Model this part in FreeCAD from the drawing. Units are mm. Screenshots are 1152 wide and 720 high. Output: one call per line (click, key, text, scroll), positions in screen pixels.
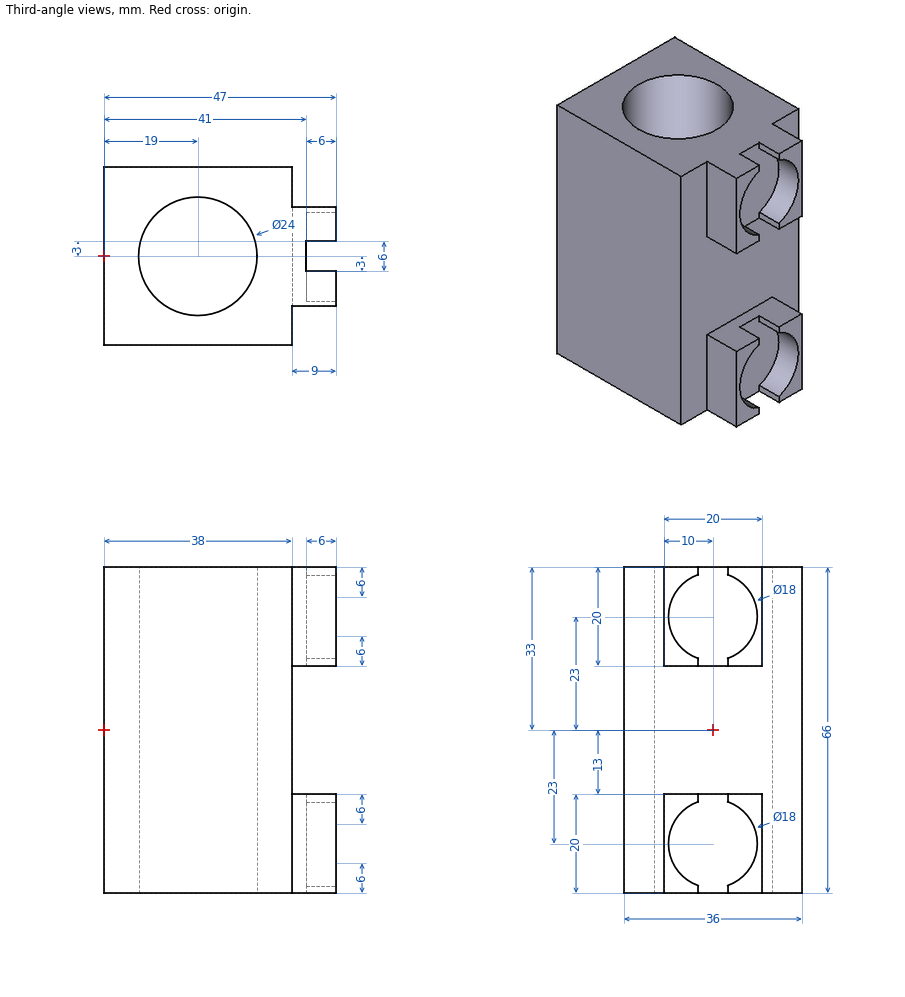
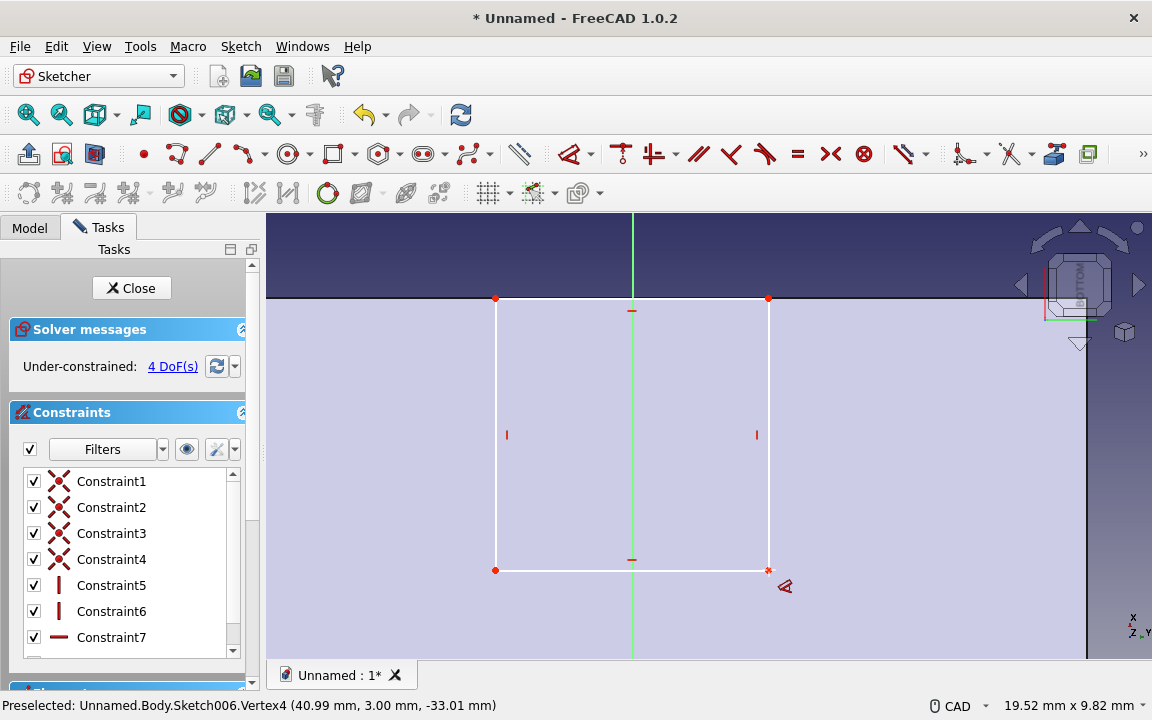
click(496, 381)
click(462, 435)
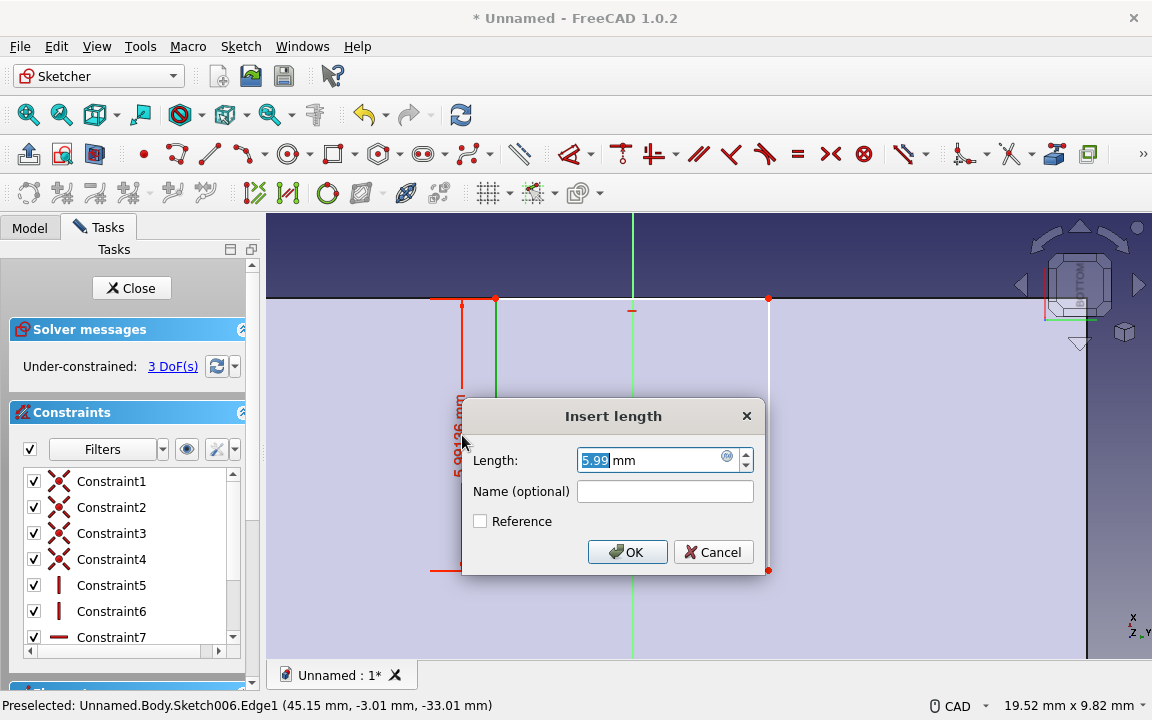
text(6)
key(Return)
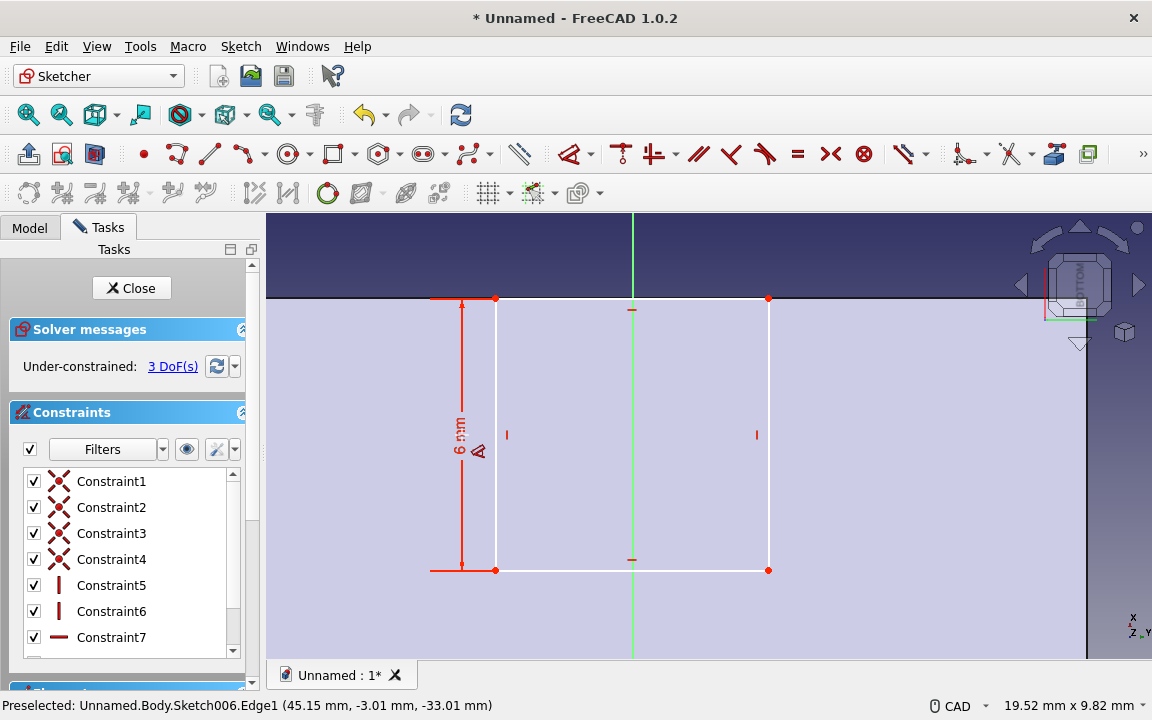
click(578, 571)
click(570, 605)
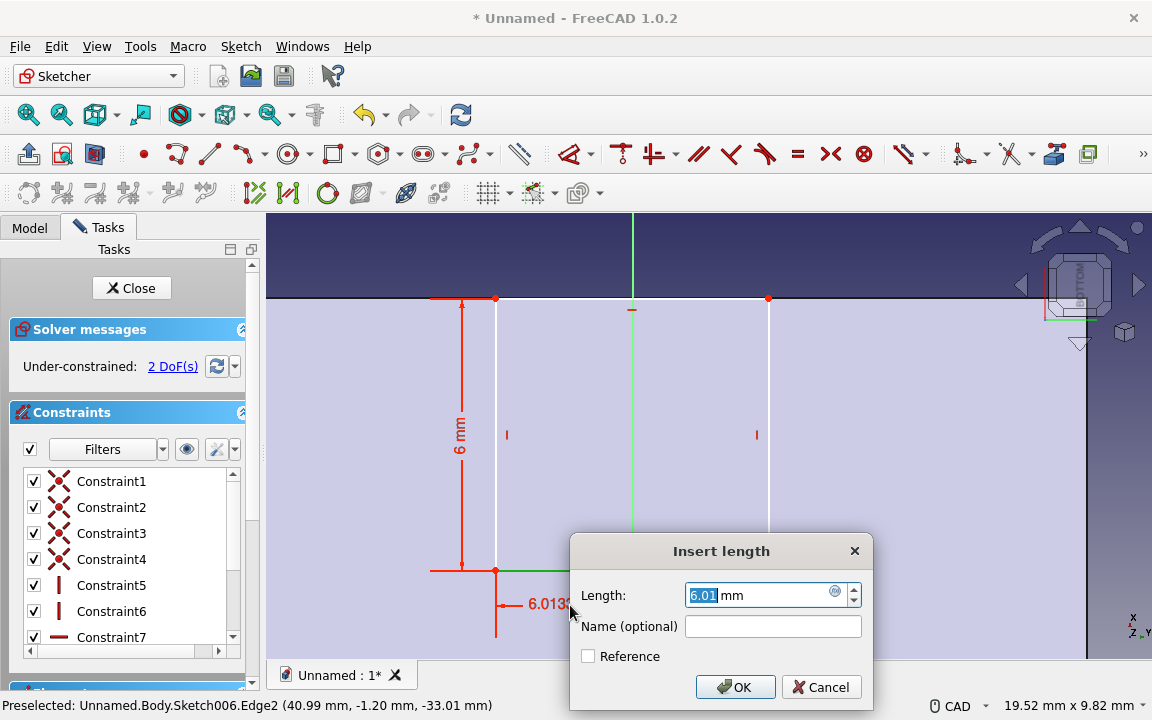
text(6)
key(Return)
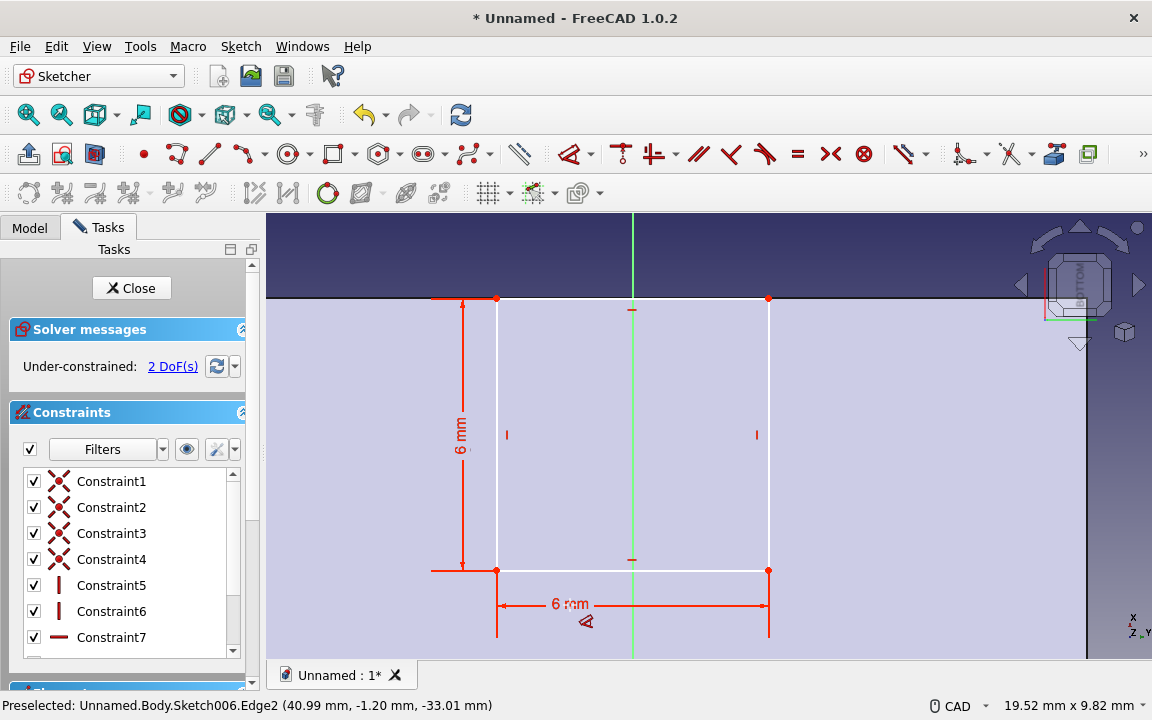
click(497, 299)
click(565, 265)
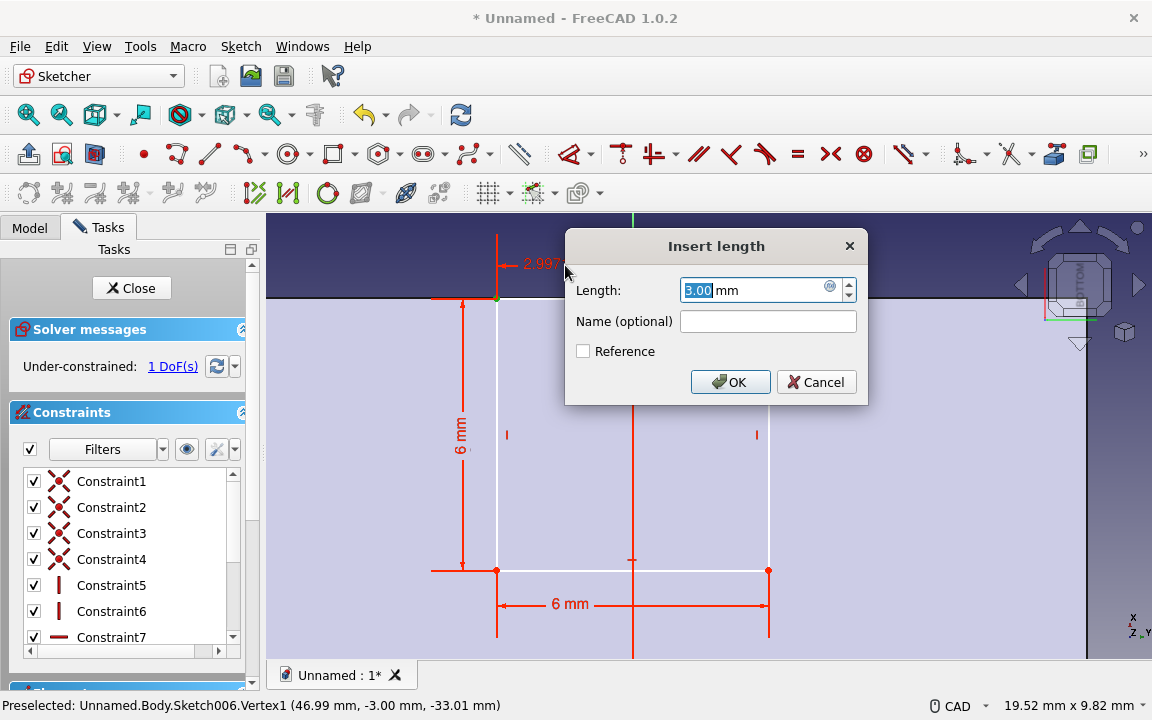
text(3)
key(Return)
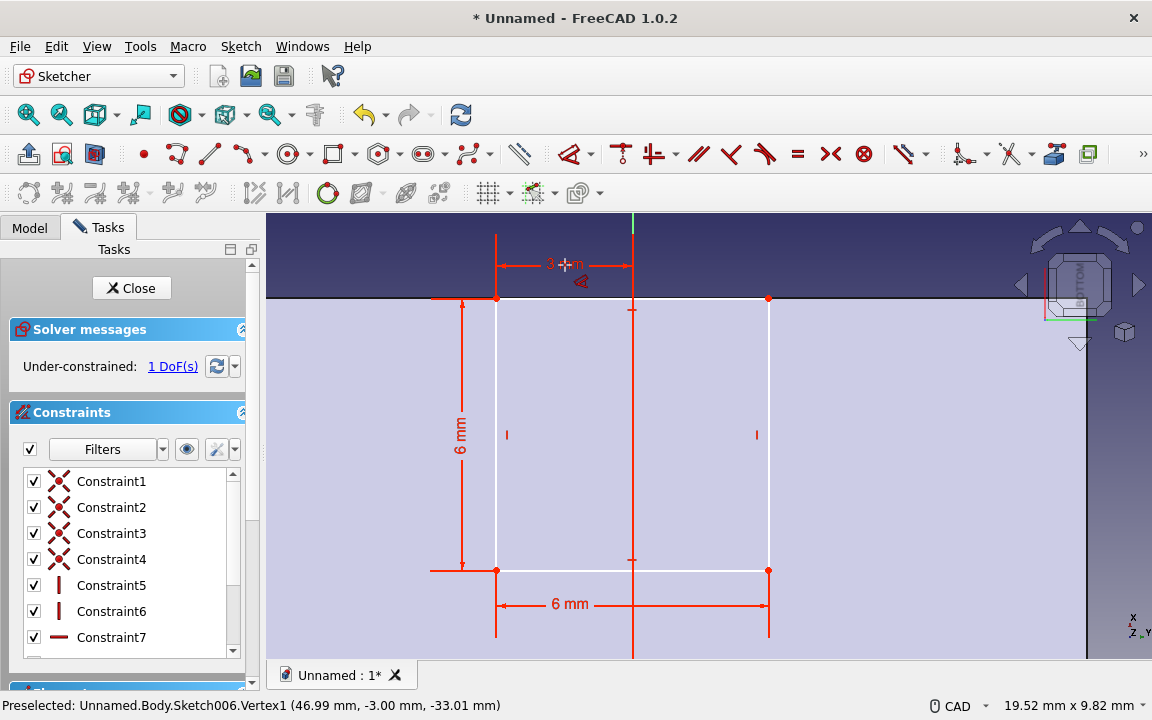
click(496, 299)
click(462, 465)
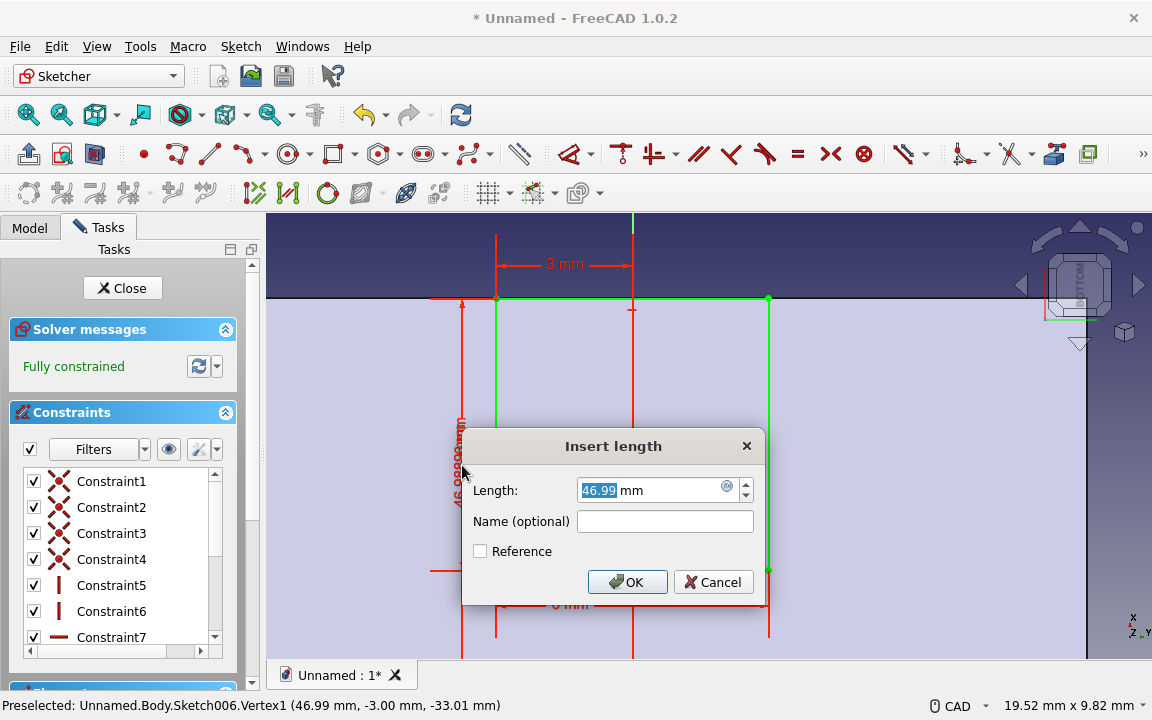
text(47)
key(Return)
key(Escape)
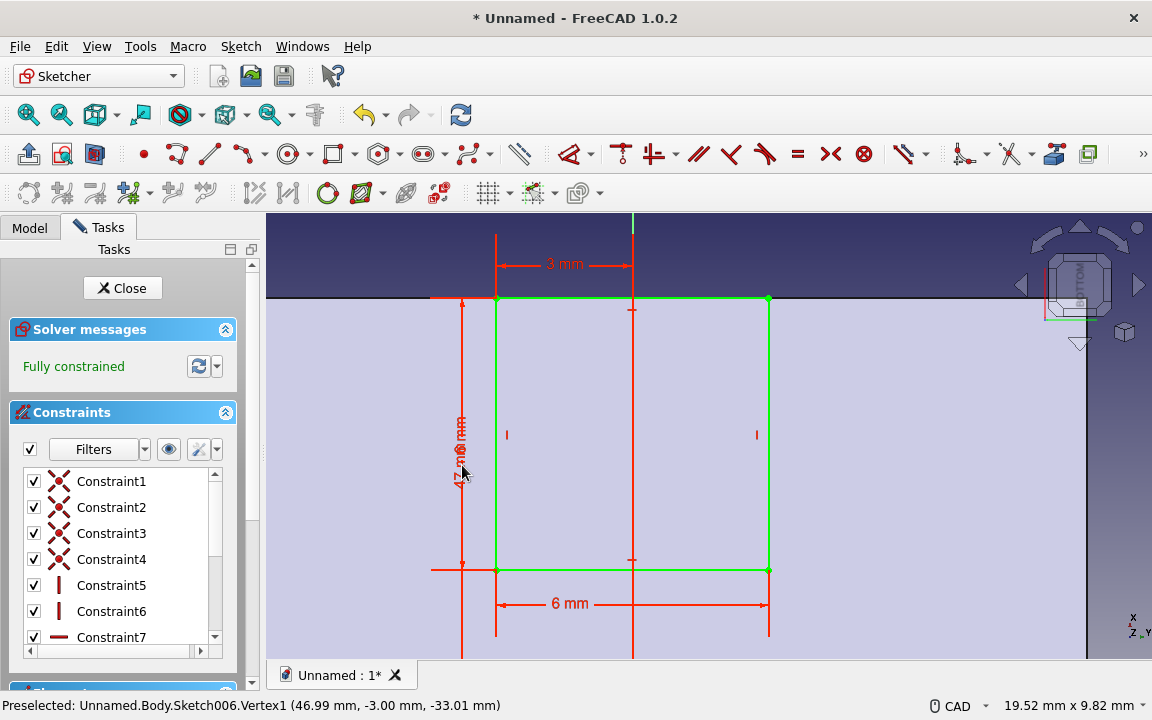
click(123, 288)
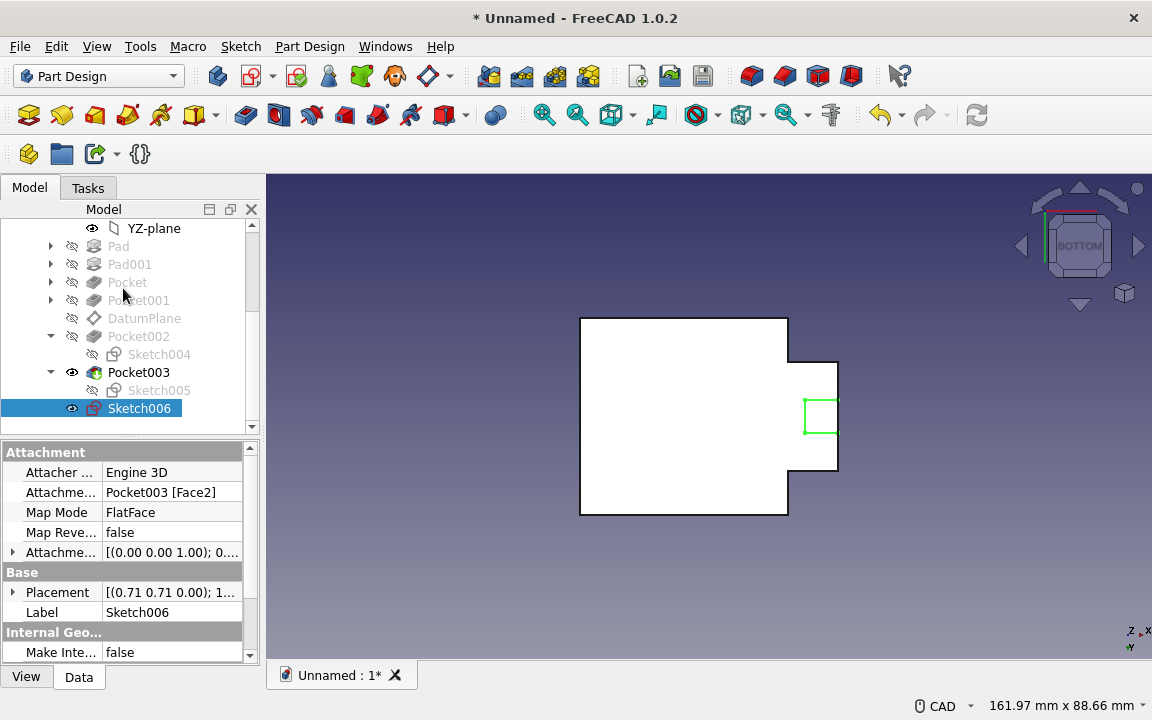
click(246, 116)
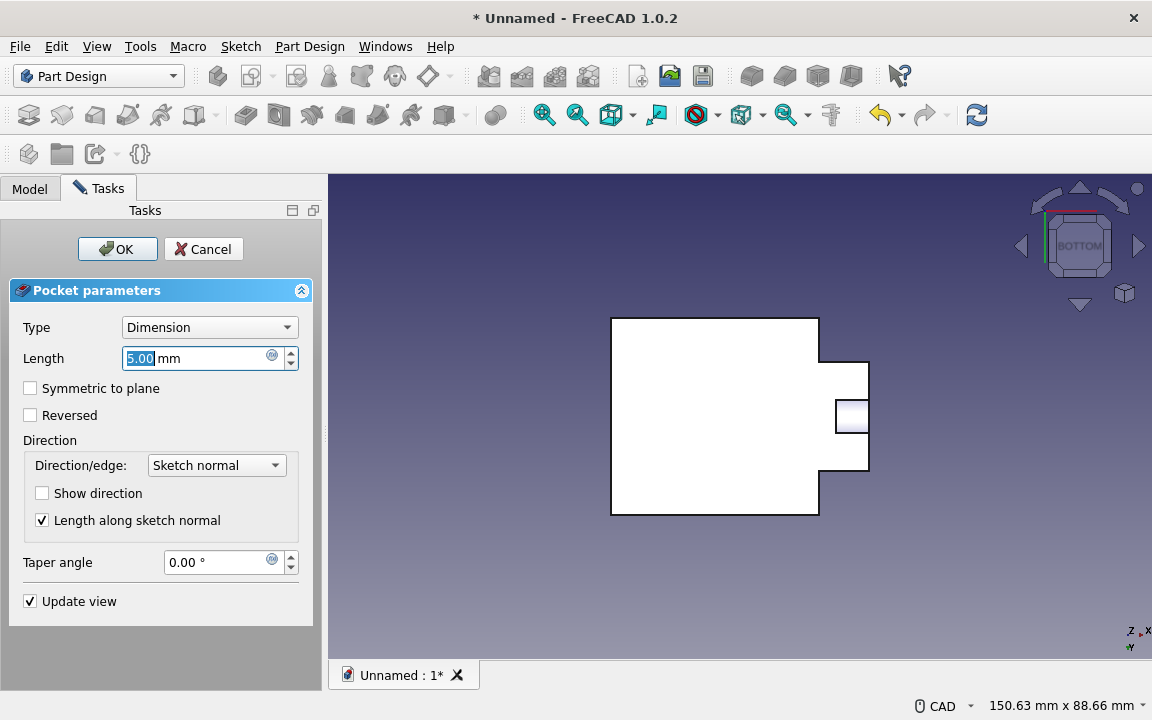
text(6)
key(Tab)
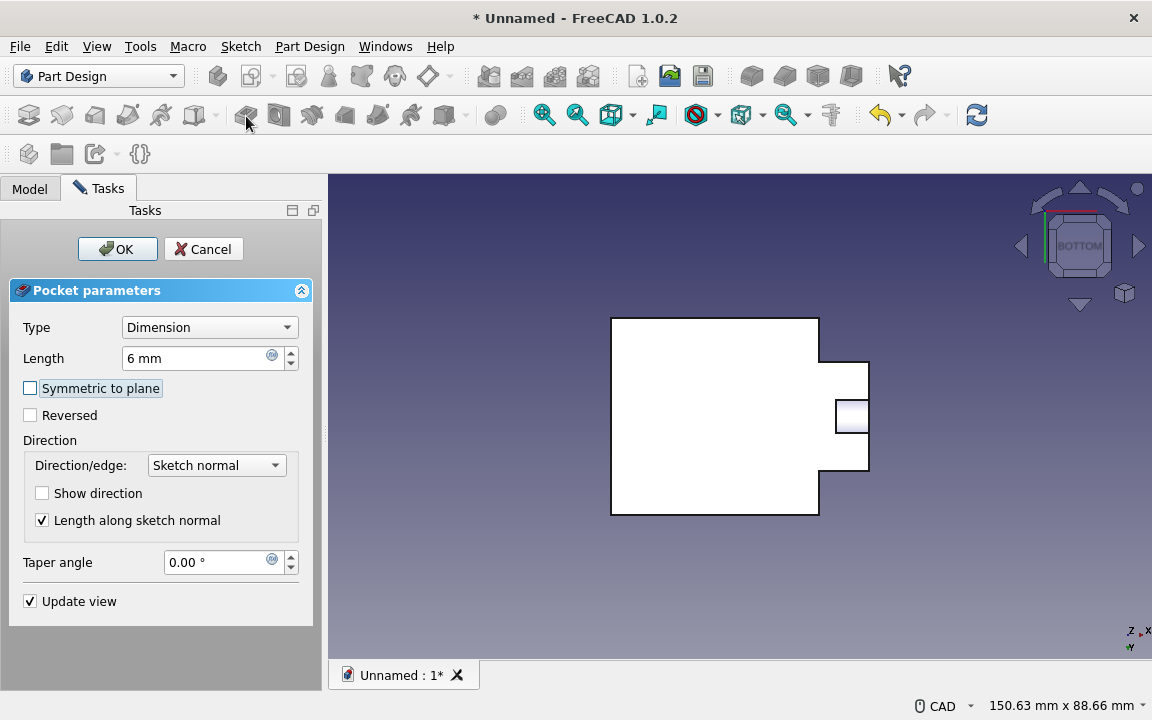
click(118, 249)